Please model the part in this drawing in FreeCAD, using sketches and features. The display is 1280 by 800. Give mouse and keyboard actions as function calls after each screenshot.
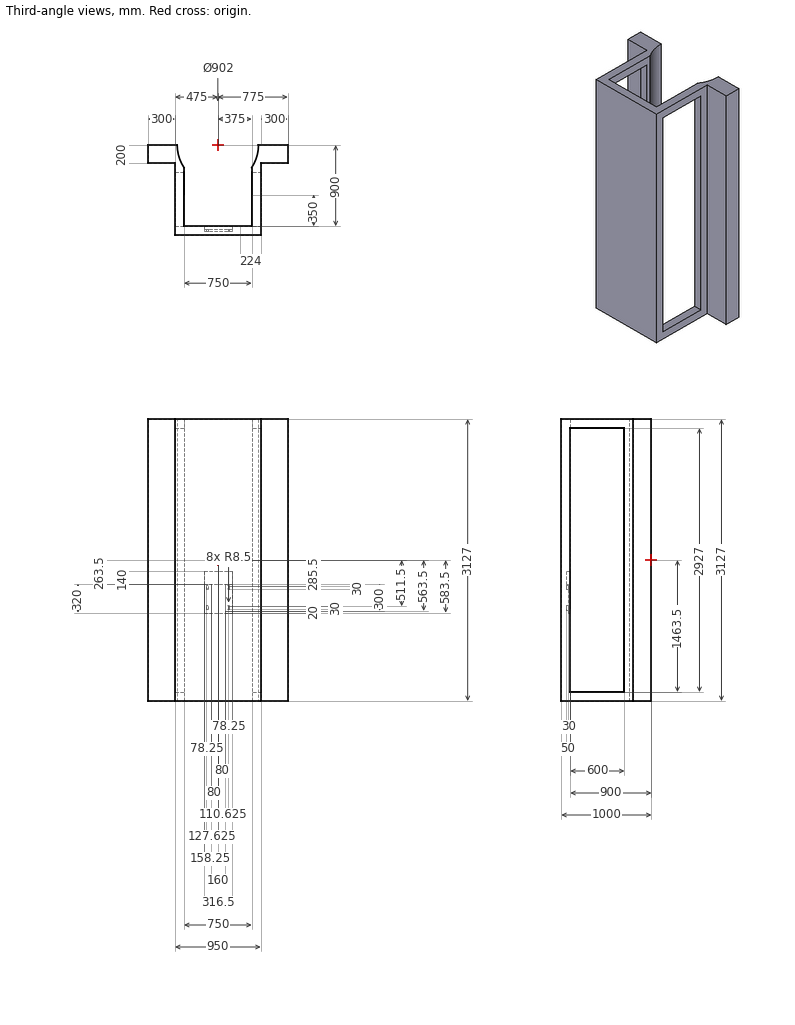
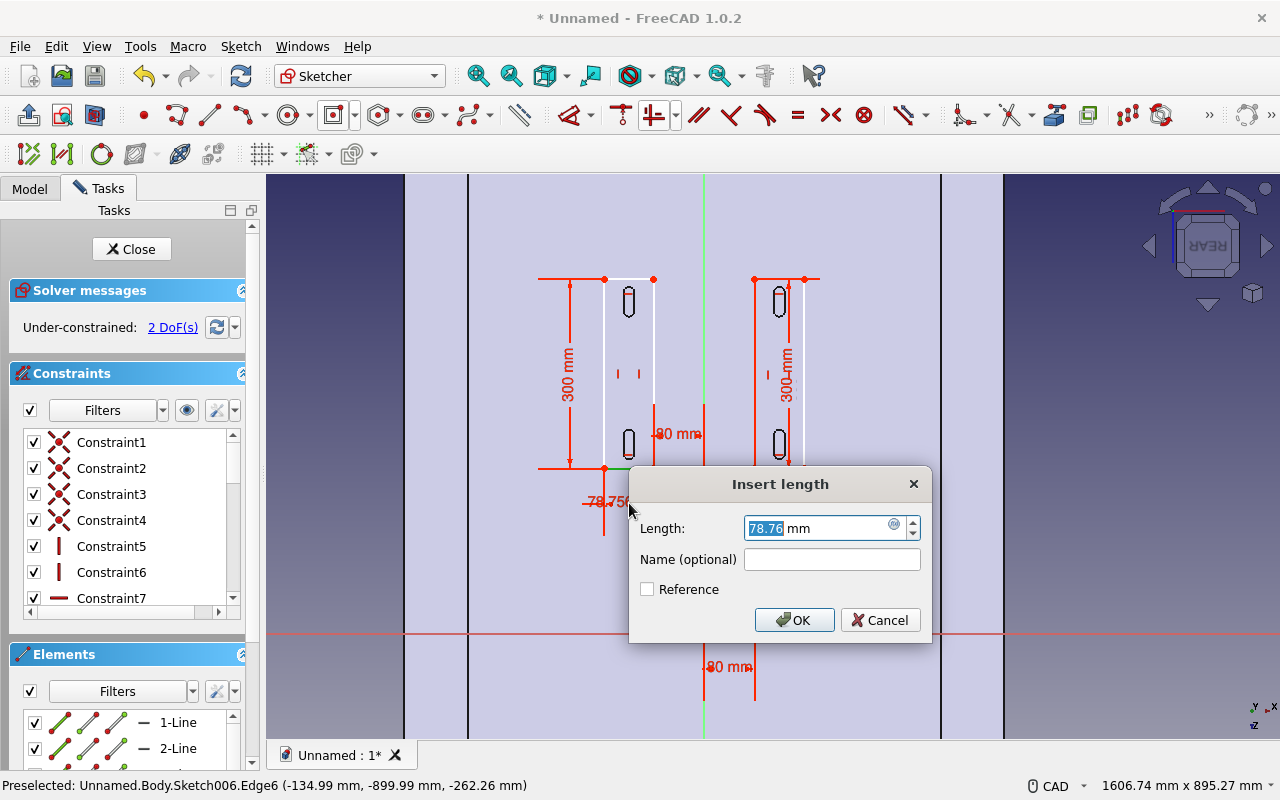
text(78.25)
key(Return)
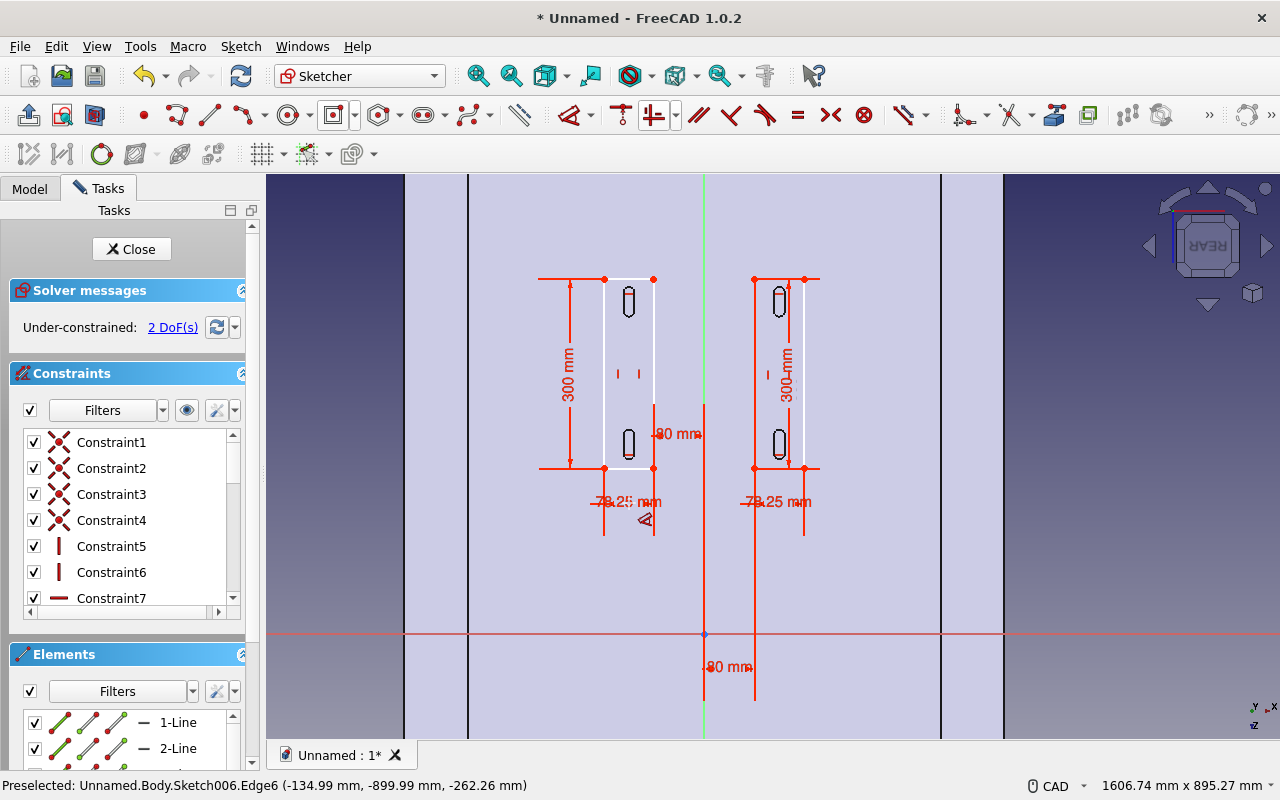
click(755, 279)
click(789, 538)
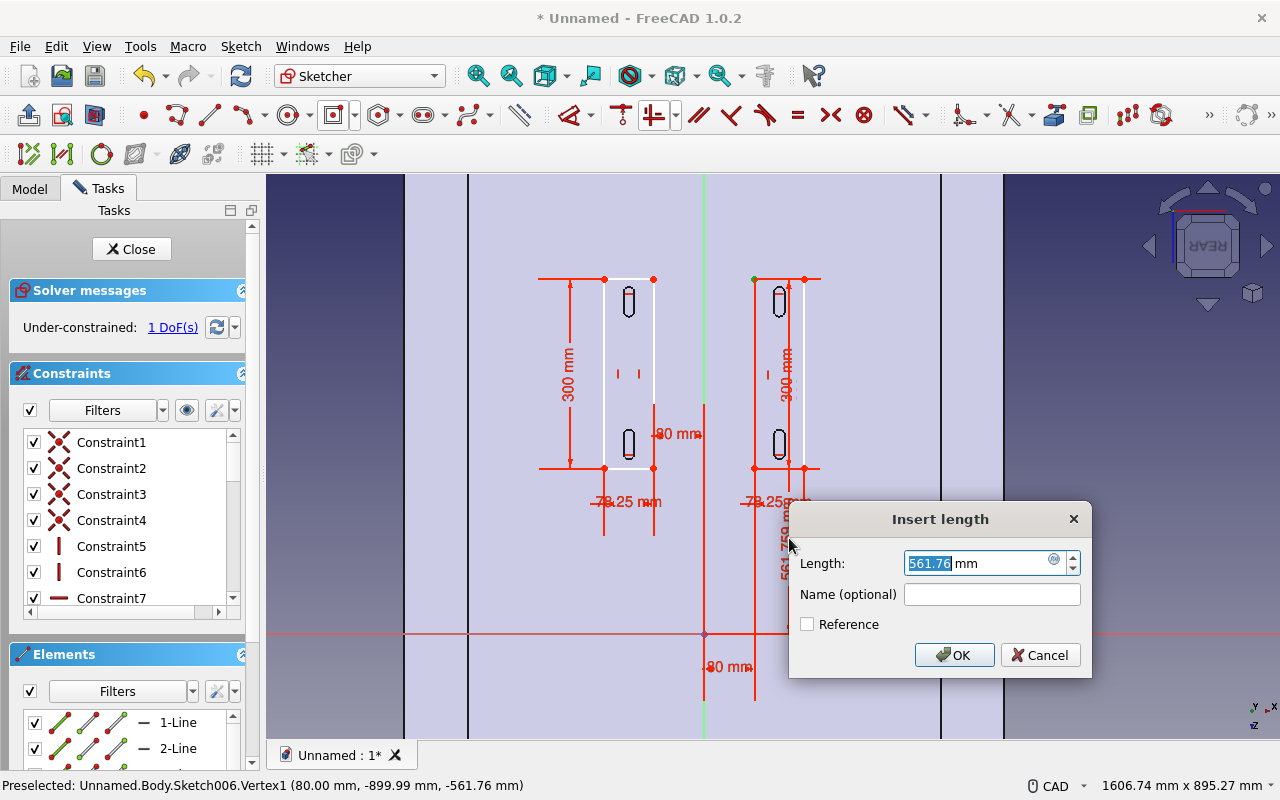
text(563.5)
key(Return)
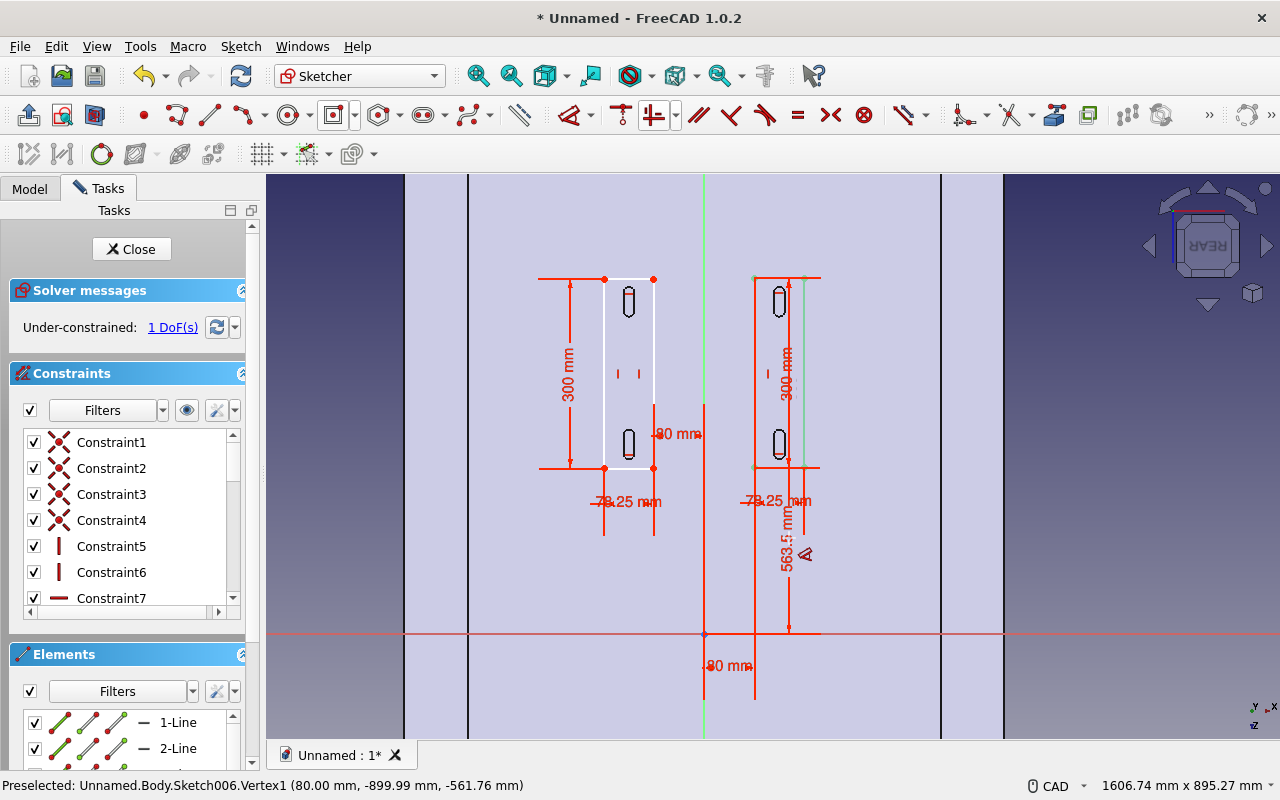
click(604, 279)
click(570, 457)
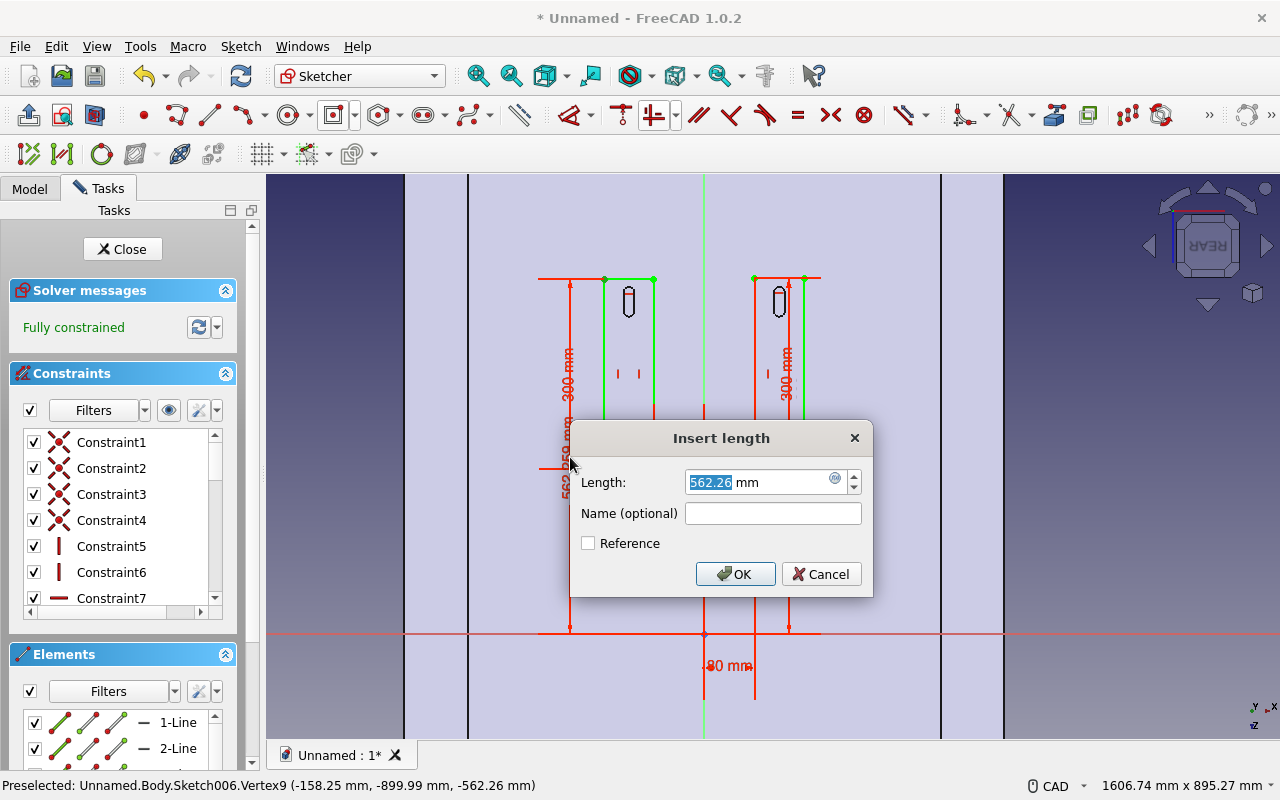
text(563.5)
key(Return)
key(Escape)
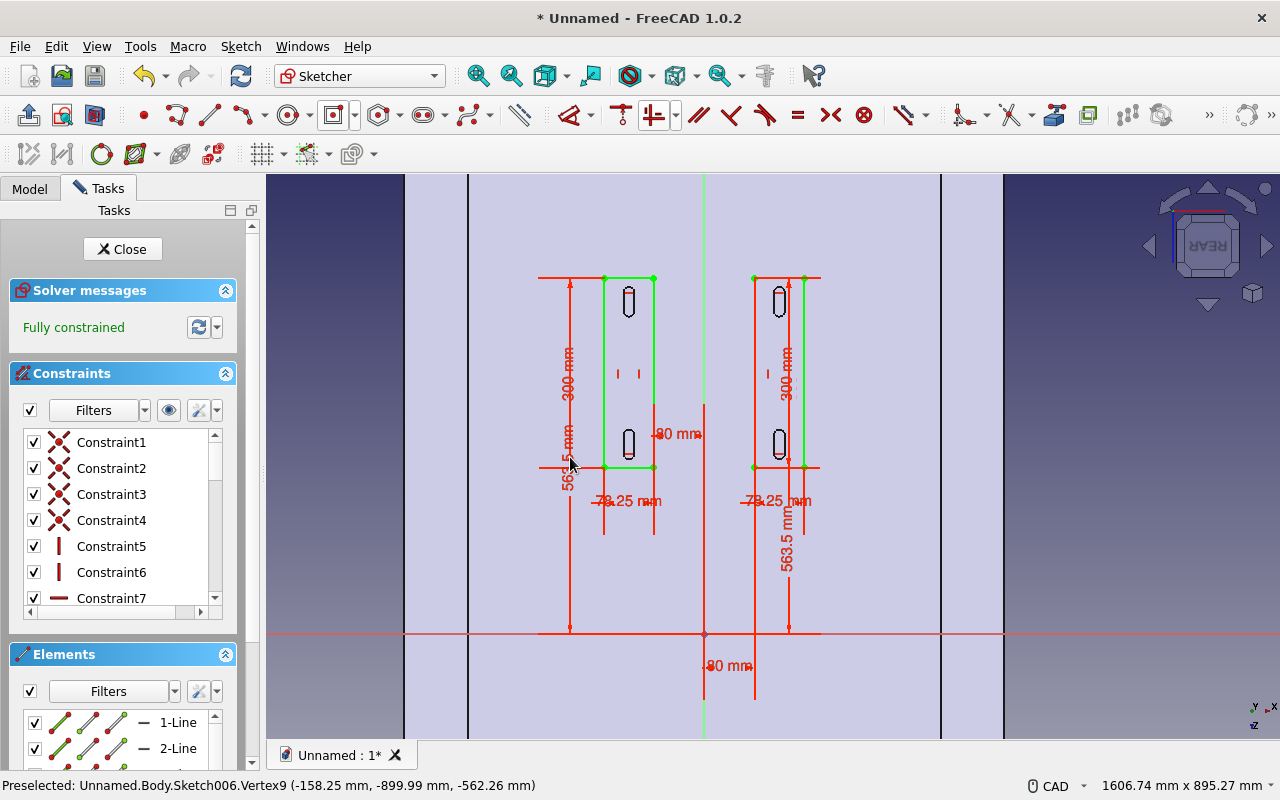
click(123, 249)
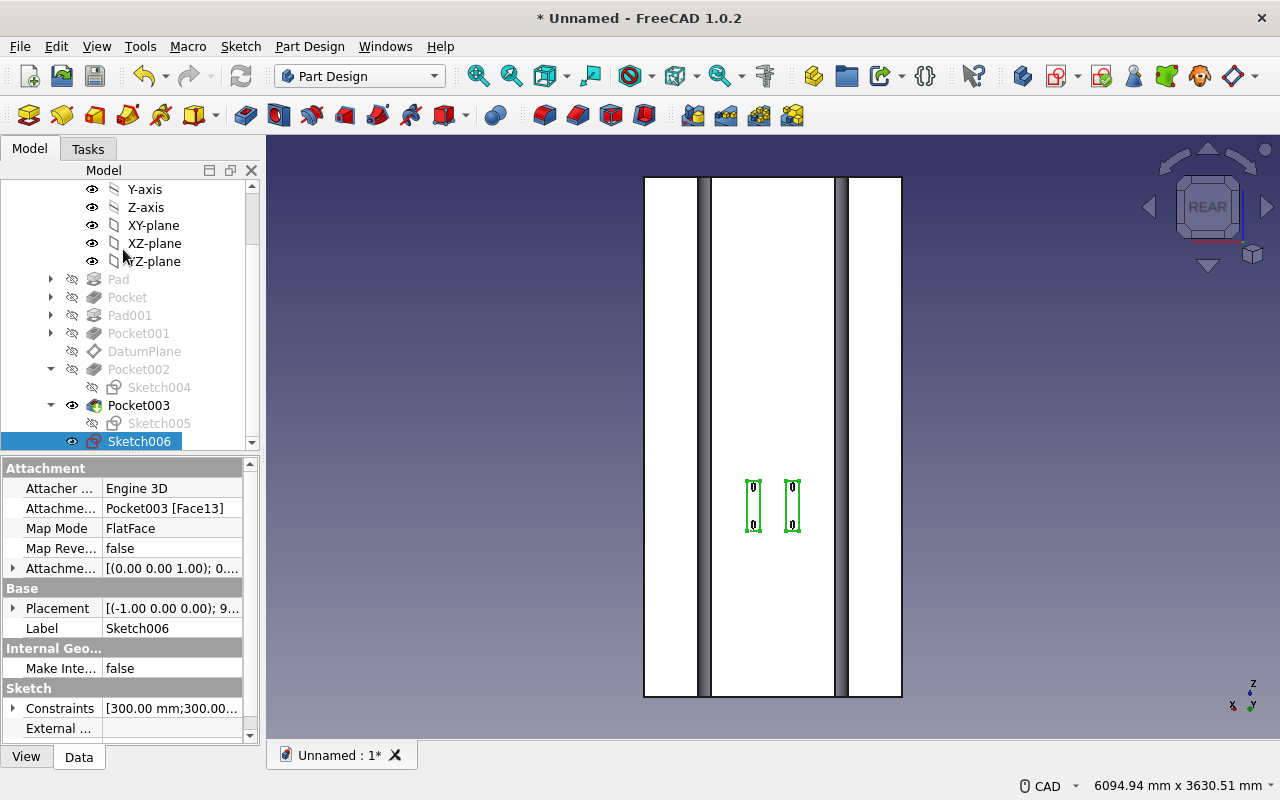
click(246, 116)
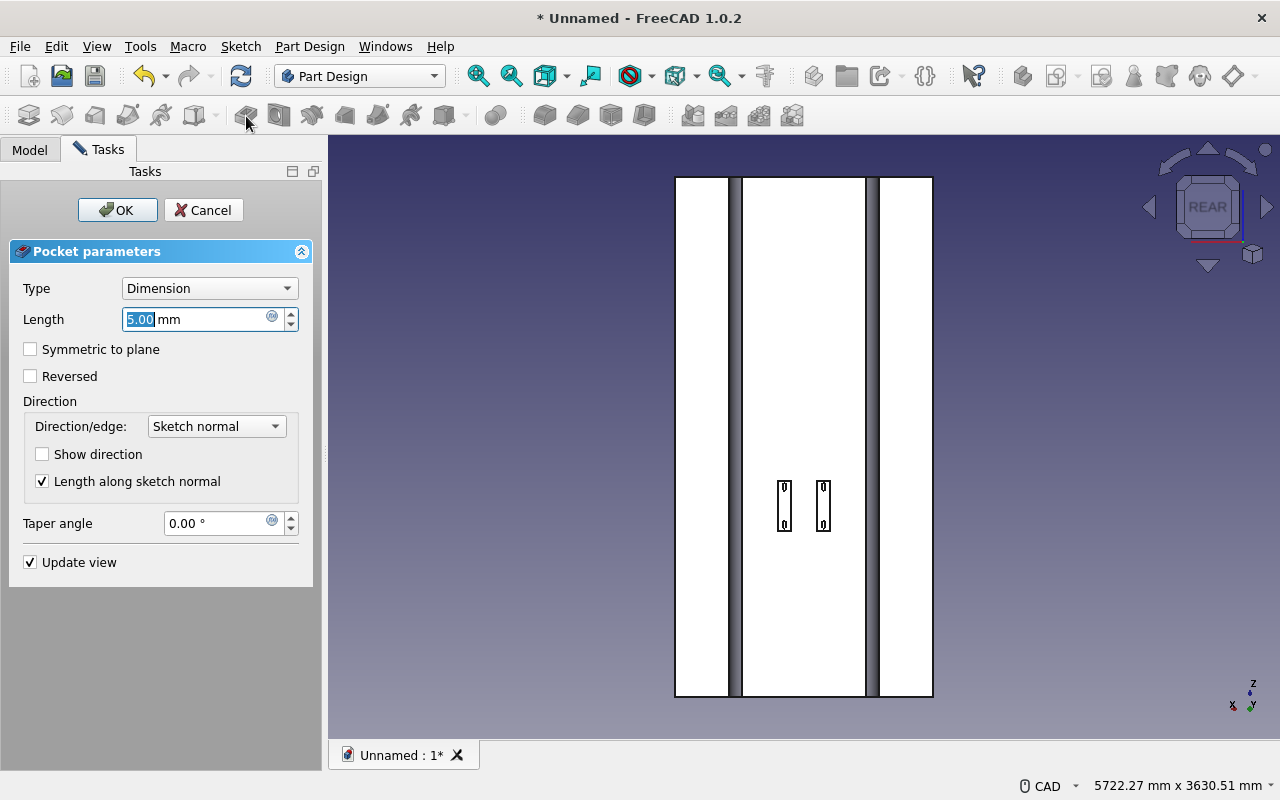
text(30)
key(Tab)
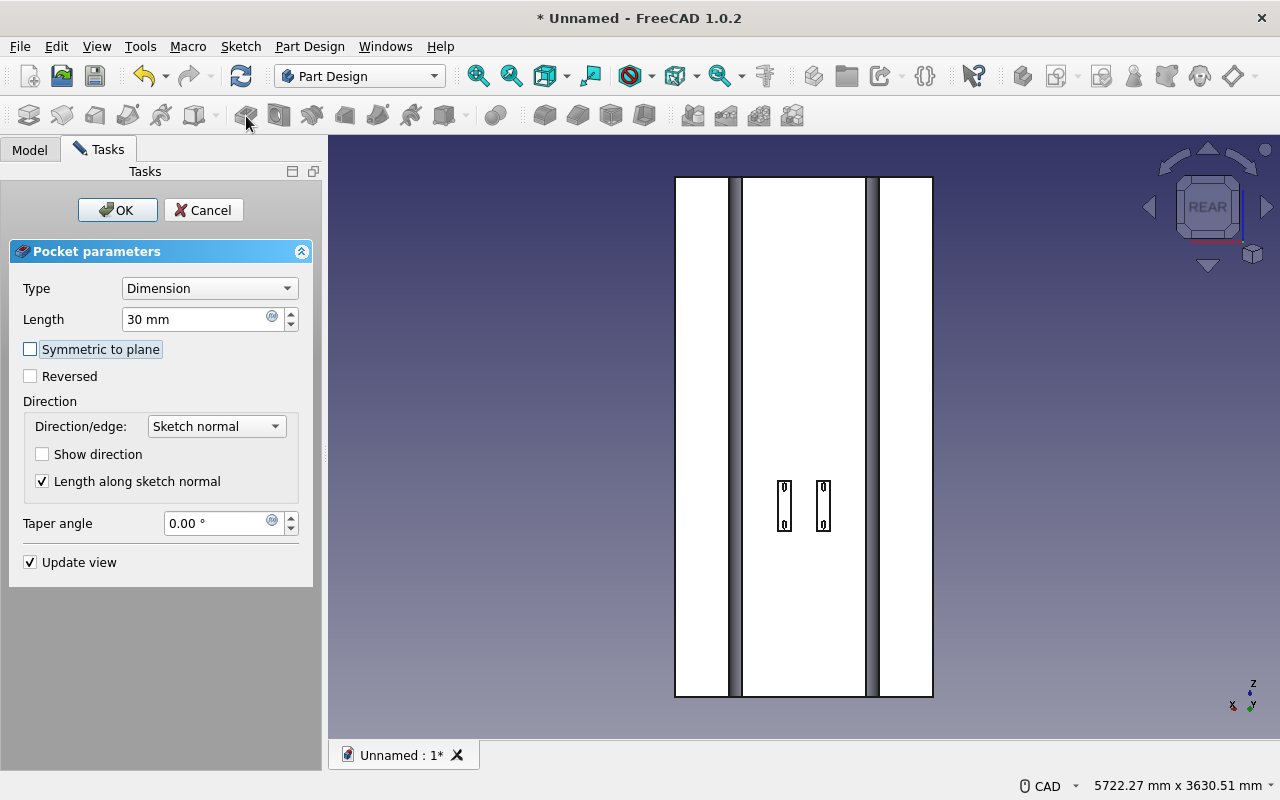
click(118, 210)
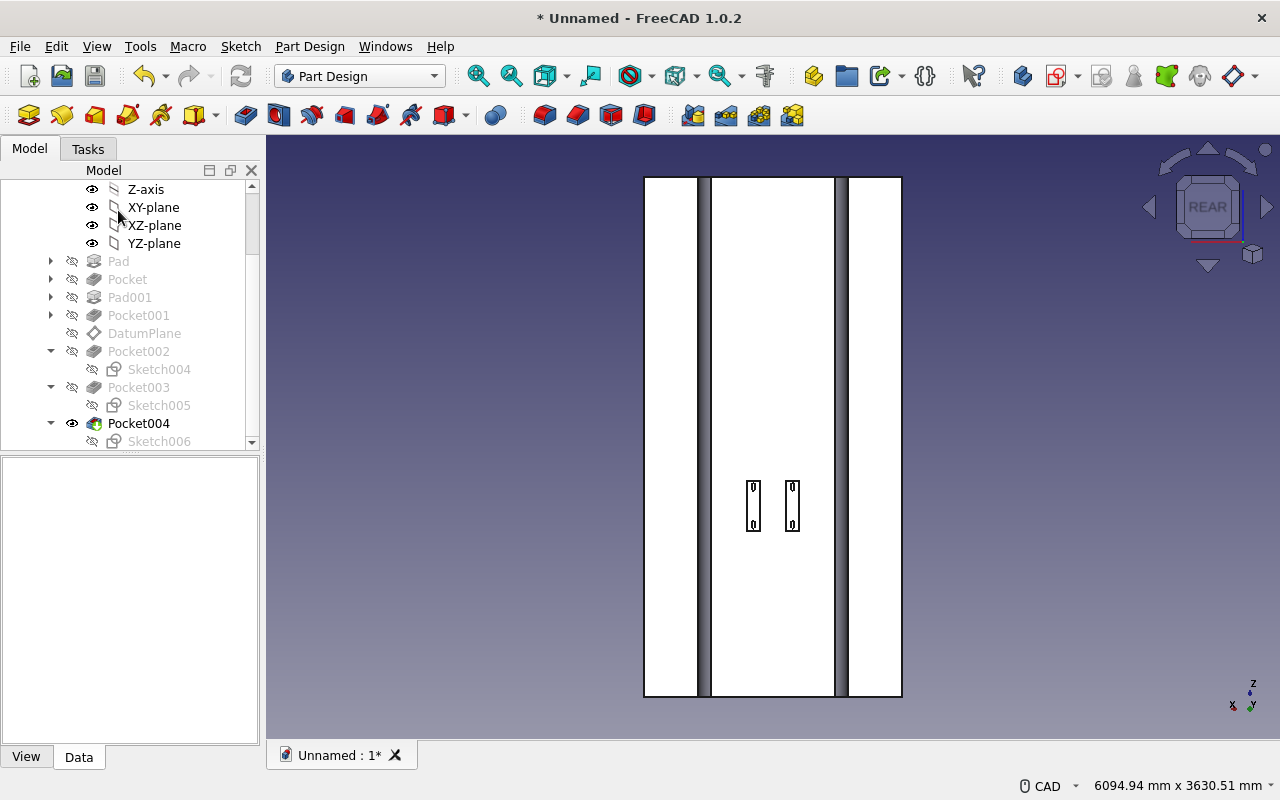
click(773, 287)